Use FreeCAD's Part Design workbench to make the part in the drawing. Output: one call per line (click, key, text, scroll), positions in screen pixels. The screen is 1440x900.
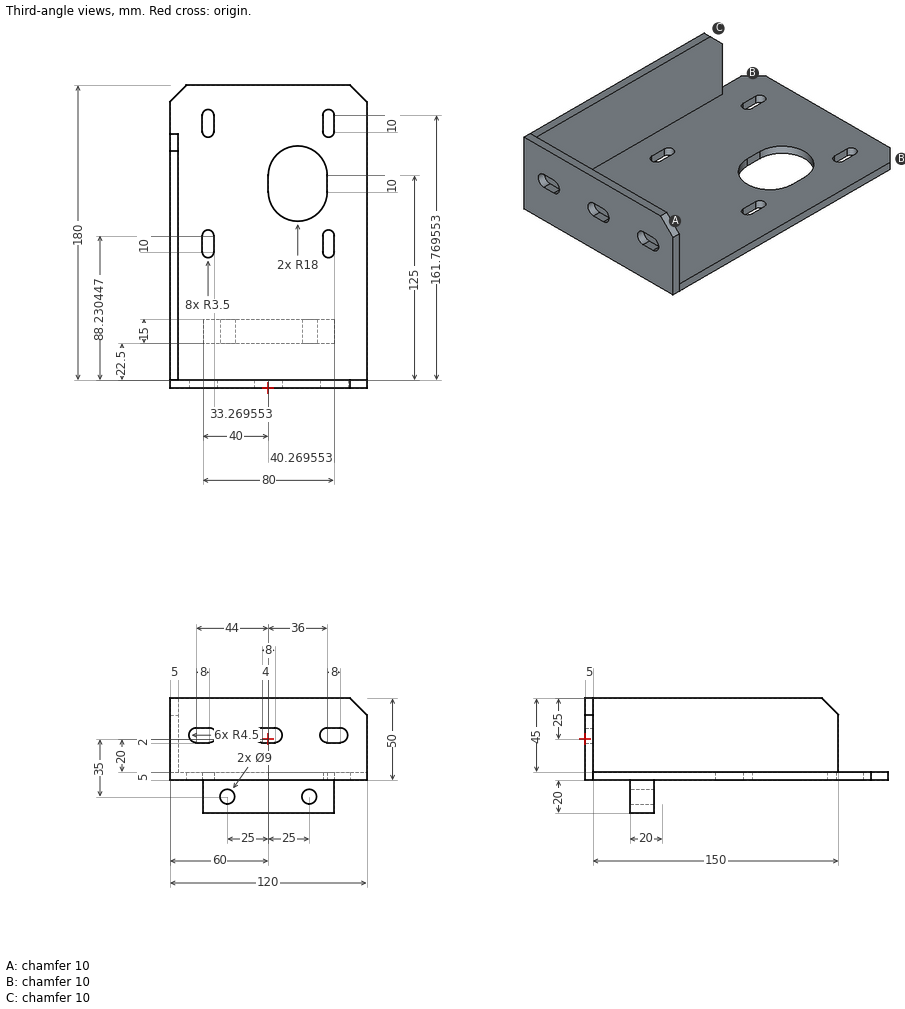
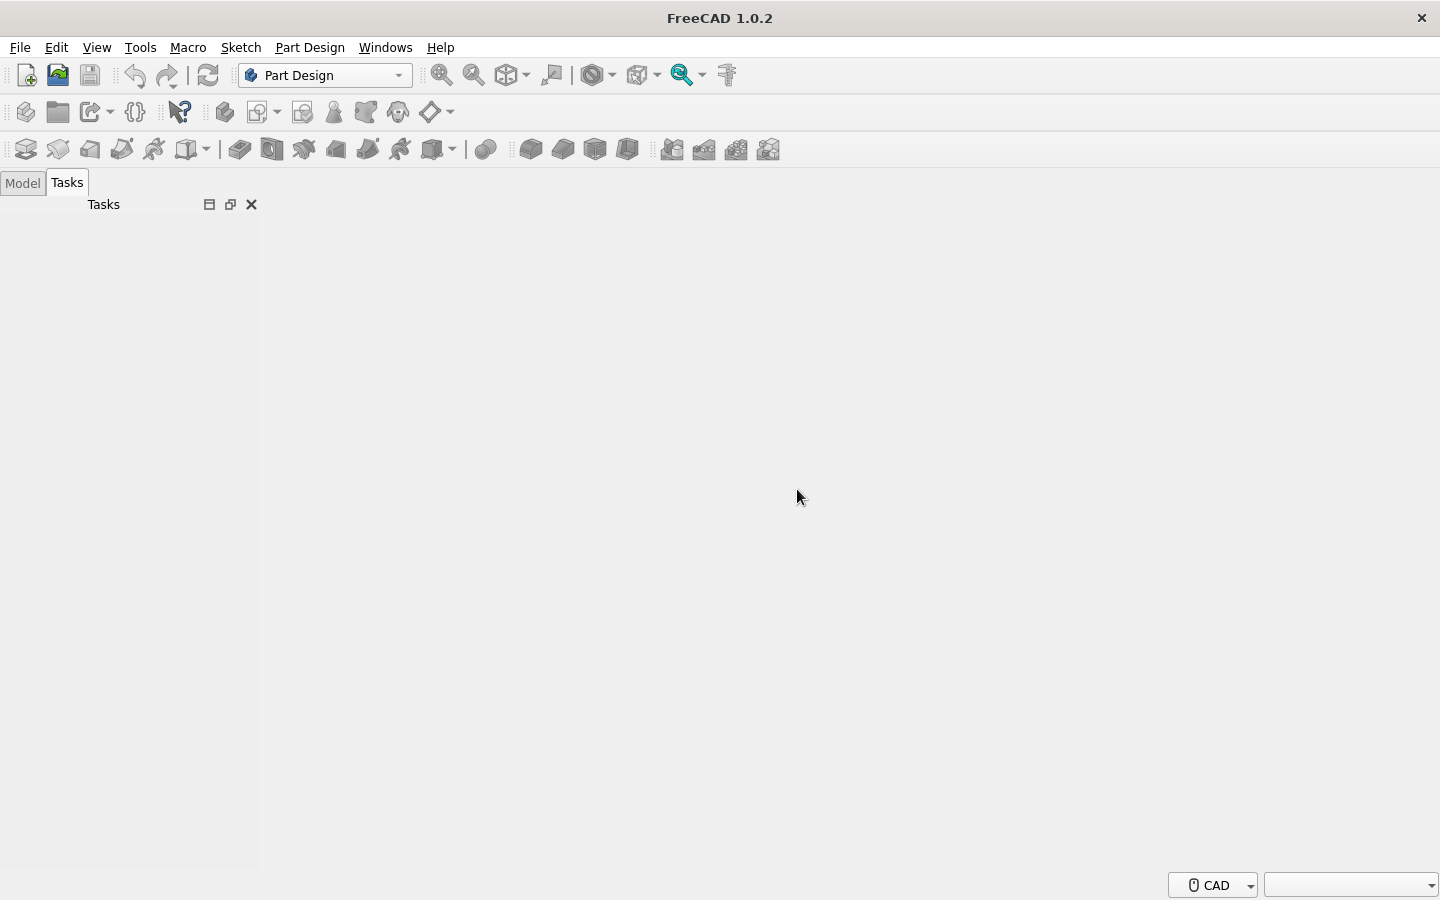
key(ctrl+n)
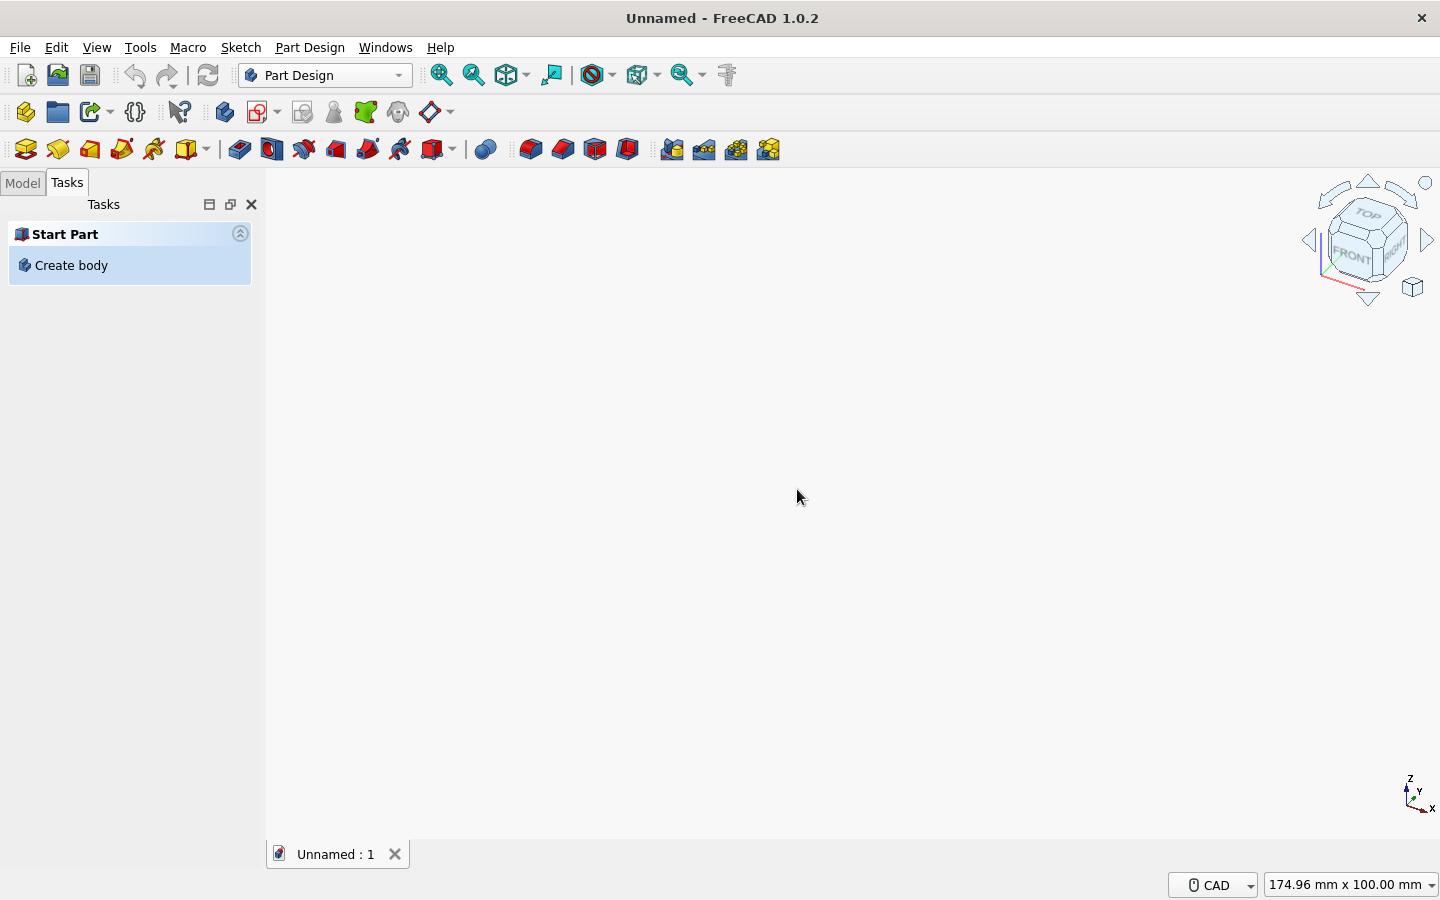
click(258, 112)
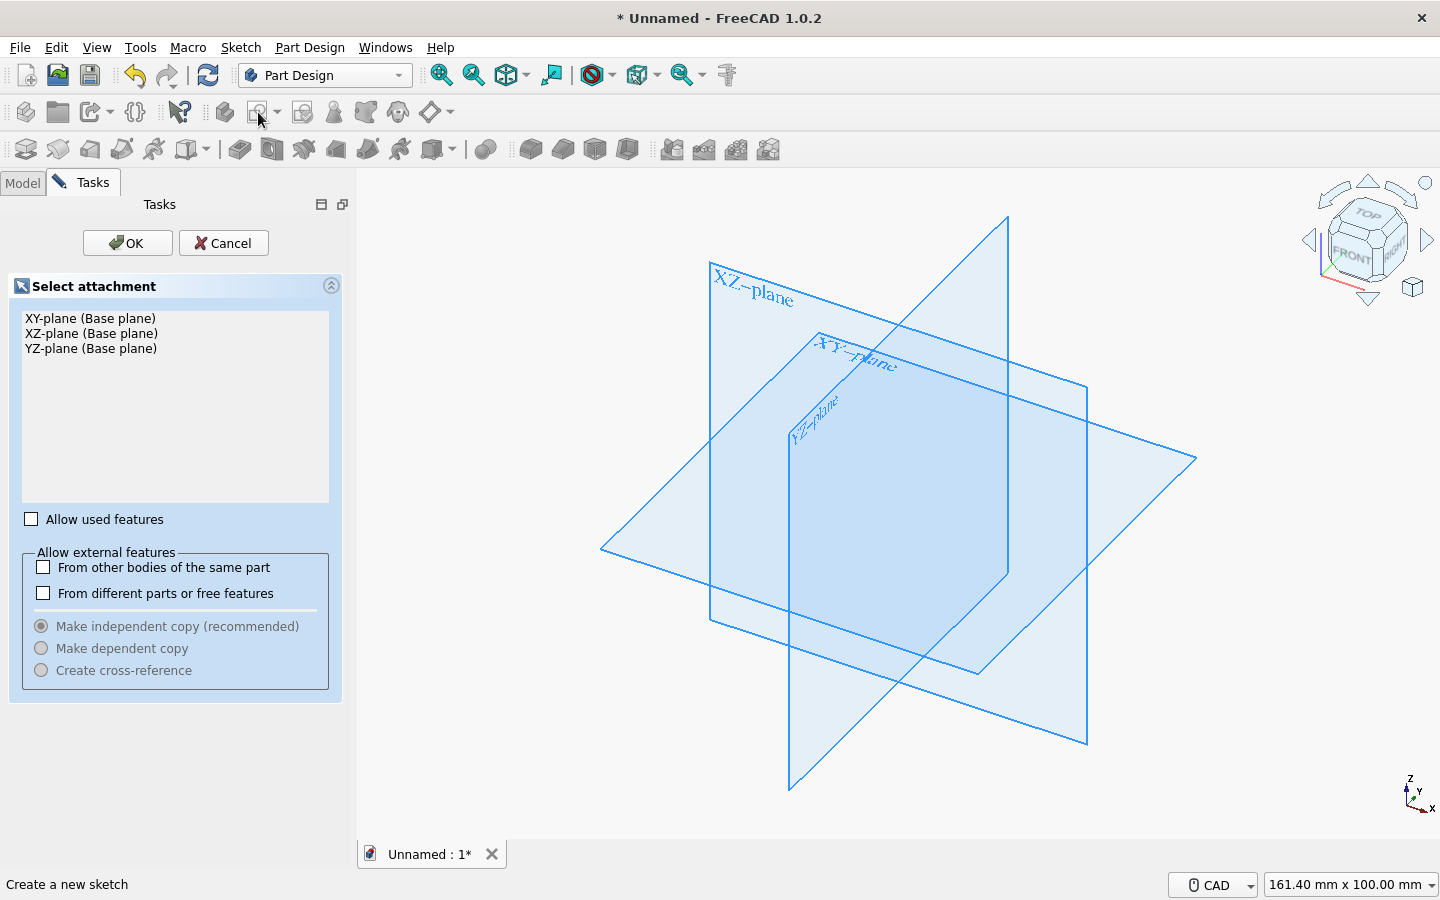
click(82, 334)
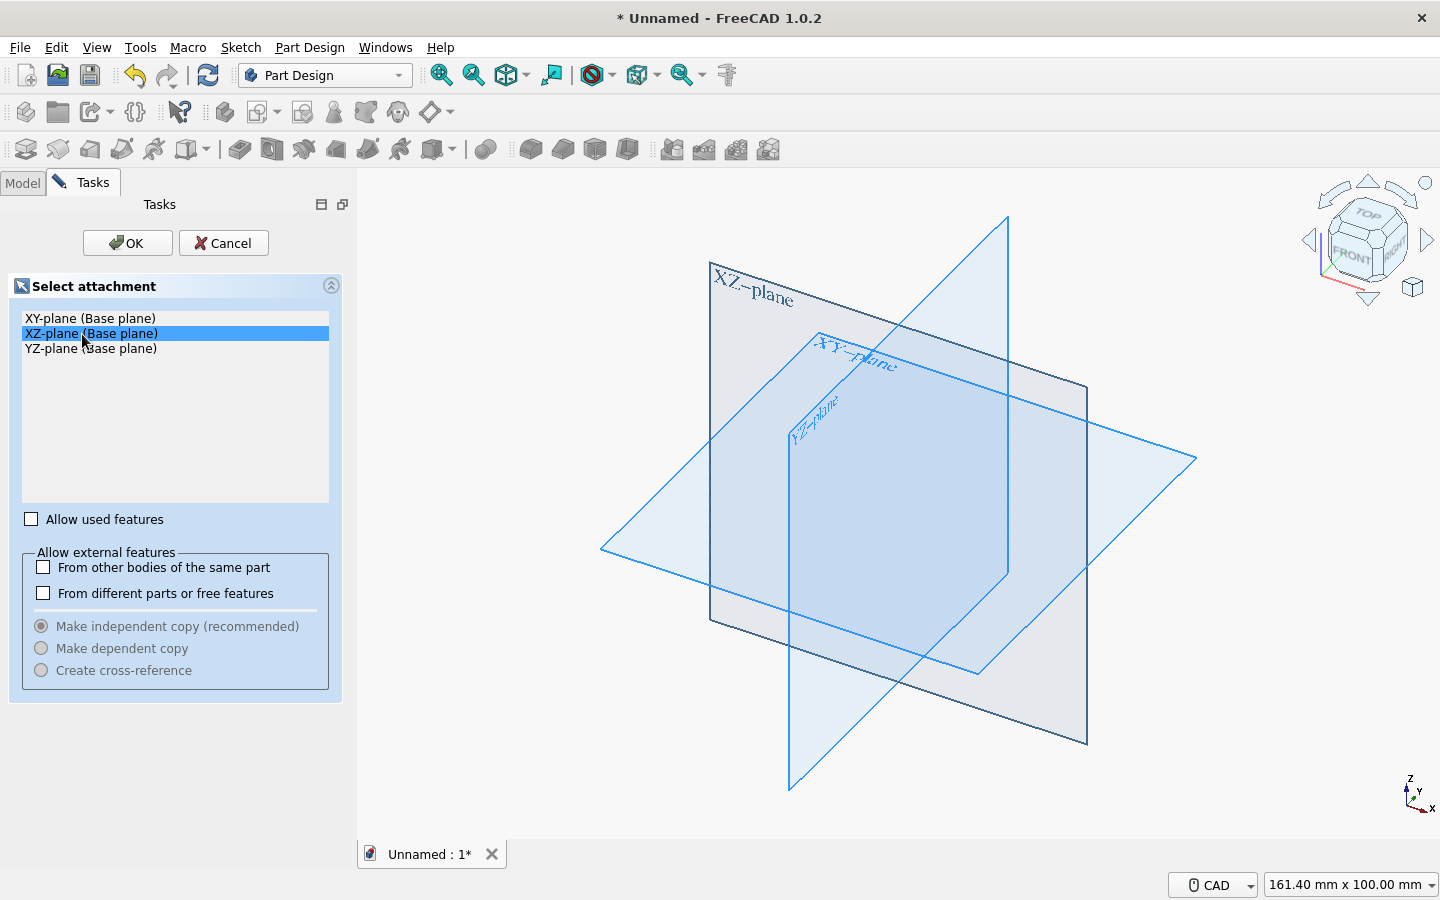
click(128, 243)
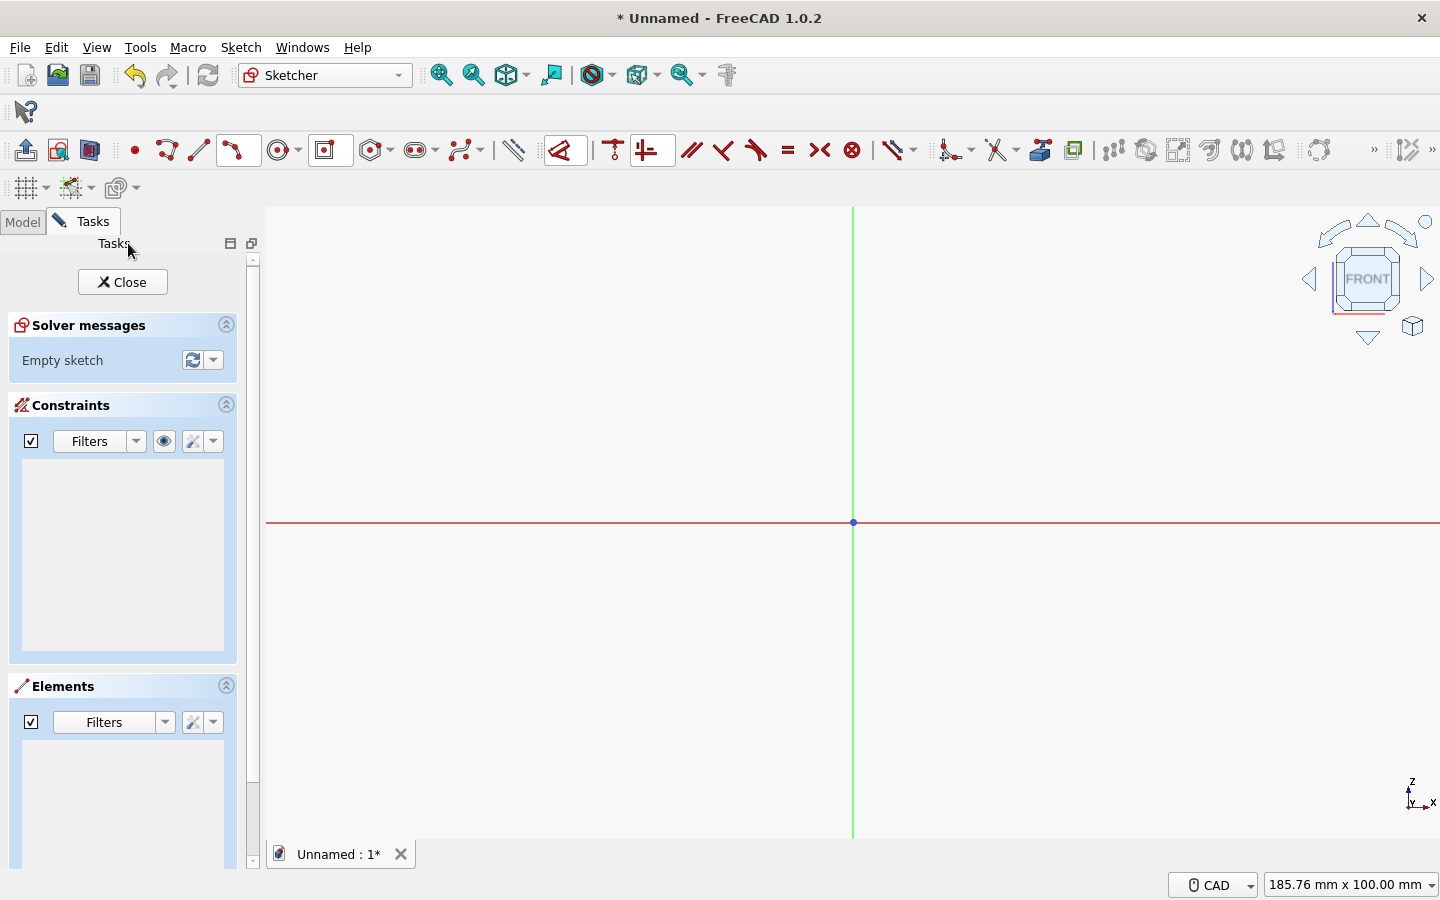
key(g)
key(v)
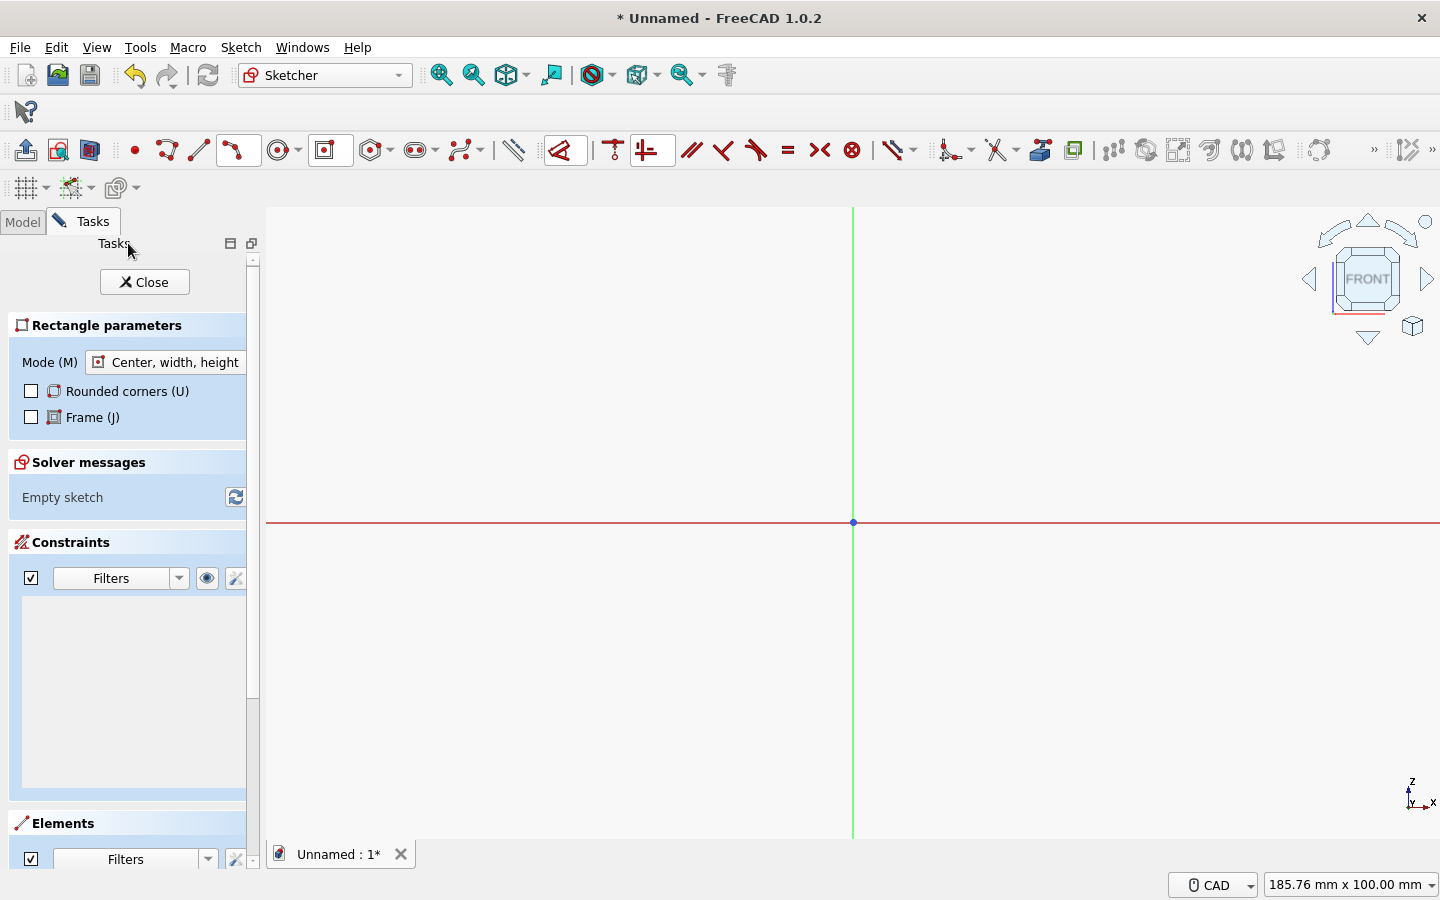
click(853, 523)
click(1232, 365)
key(Escape)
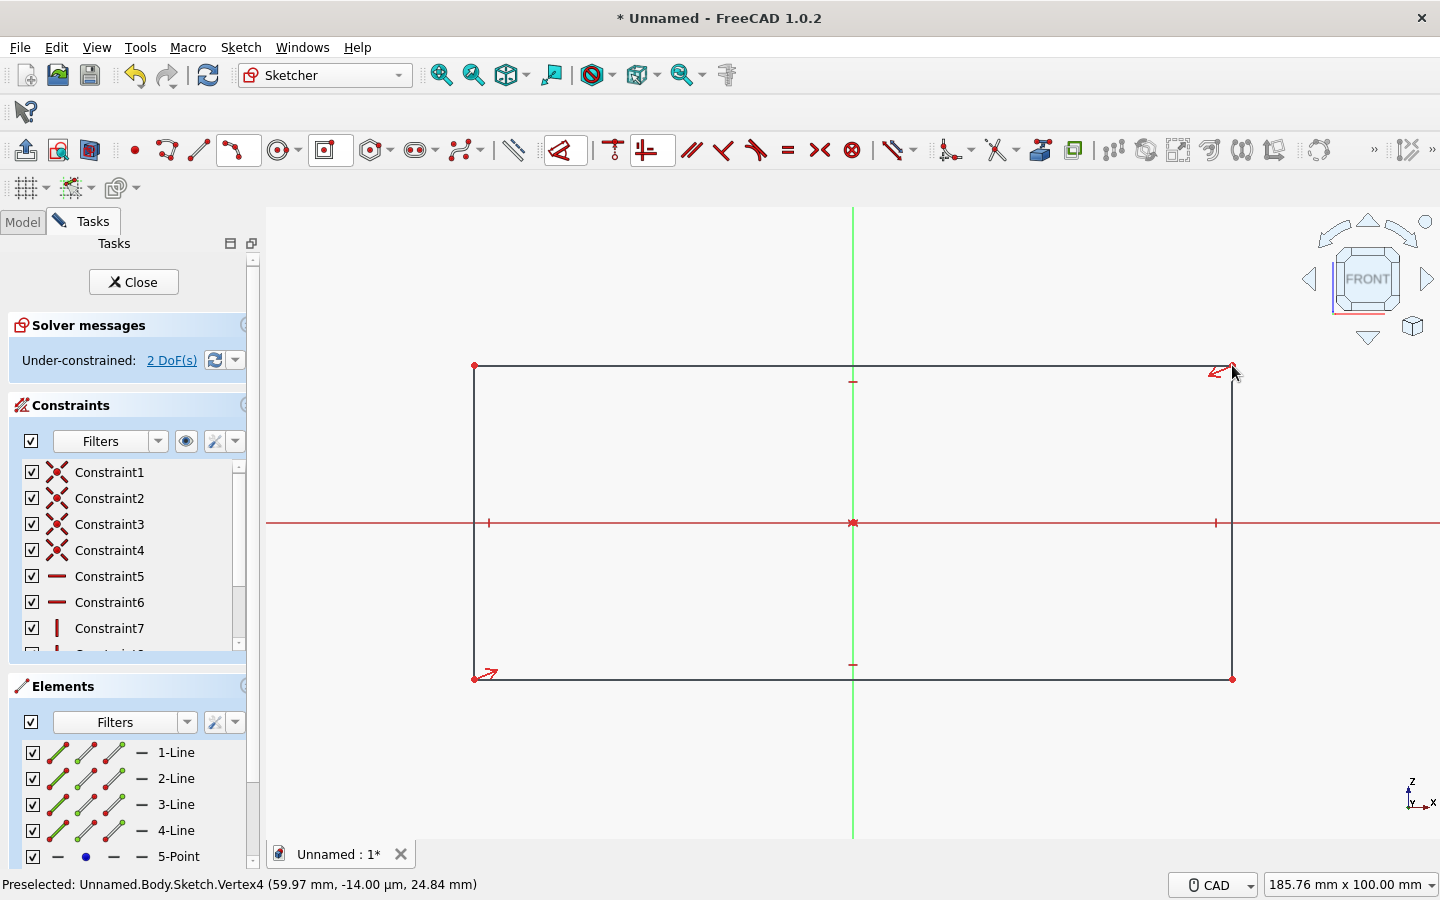
click(560, 150)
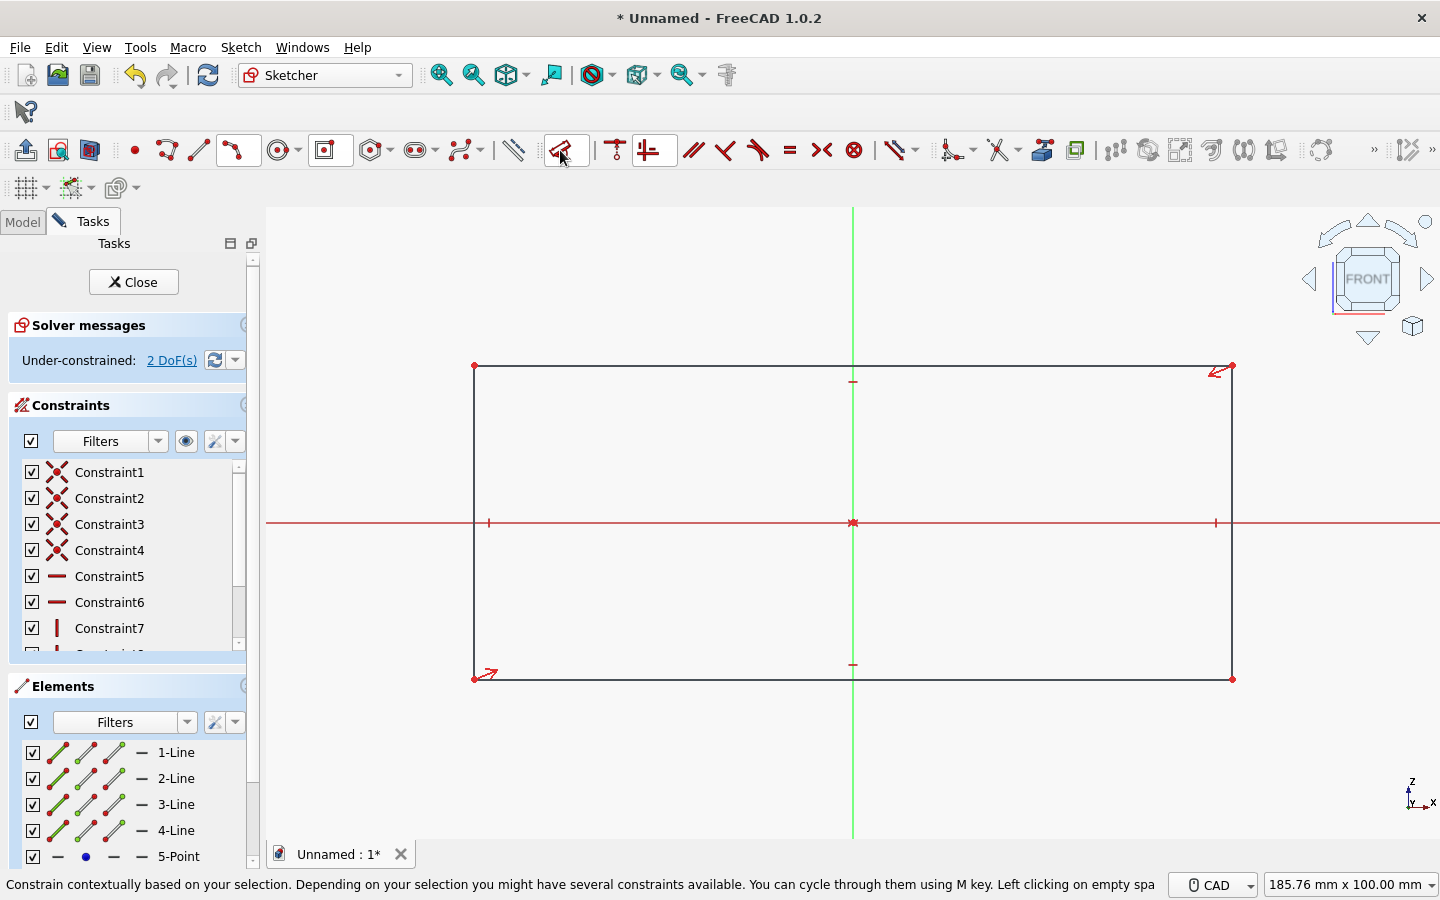
click(1232, 586)
click(1266, 451)